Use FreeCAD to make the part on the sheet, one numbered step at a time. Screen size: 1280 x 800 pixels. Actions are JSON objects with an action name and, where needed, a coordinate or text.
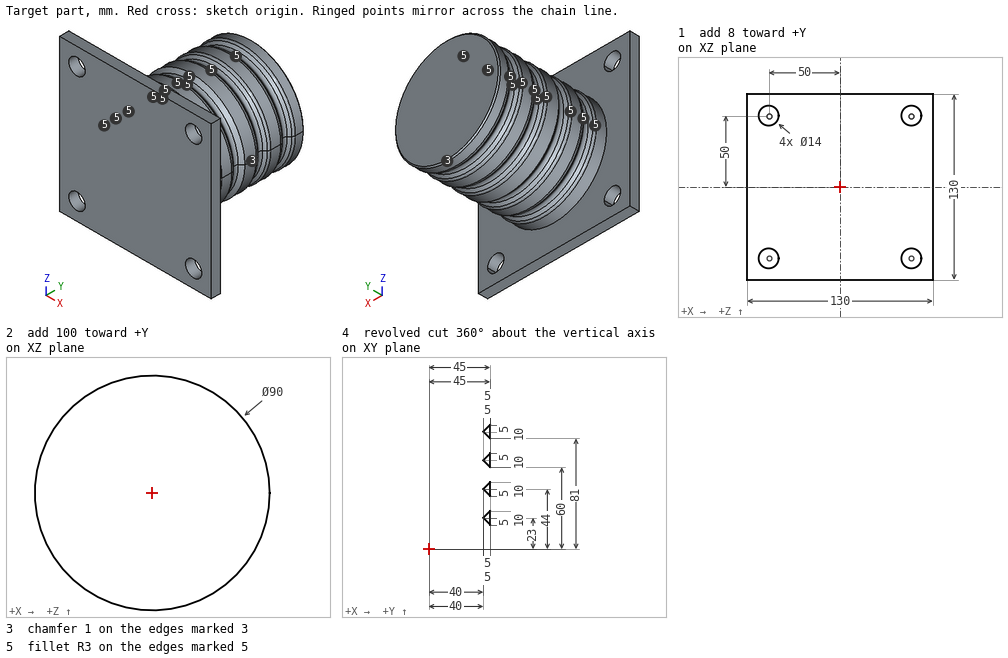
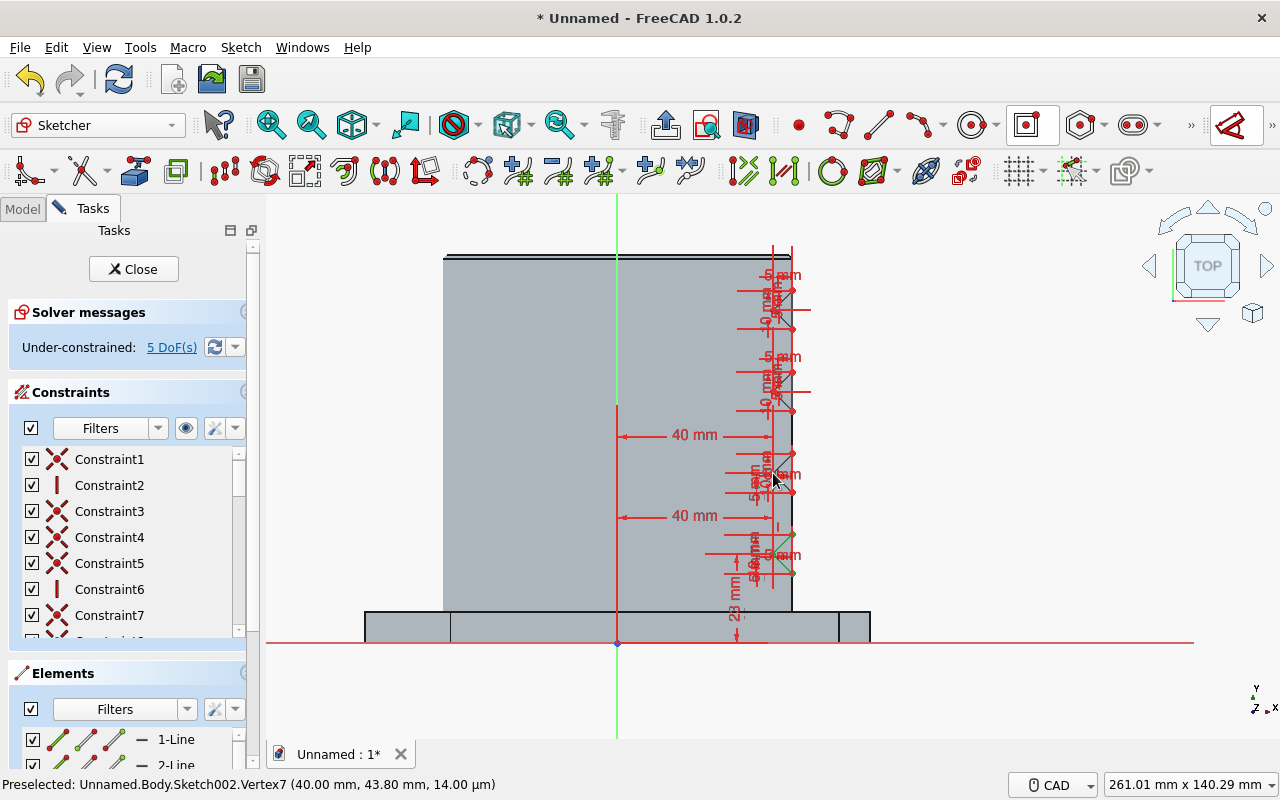
{"action": "left_click", "coordinate": [1258, 126]}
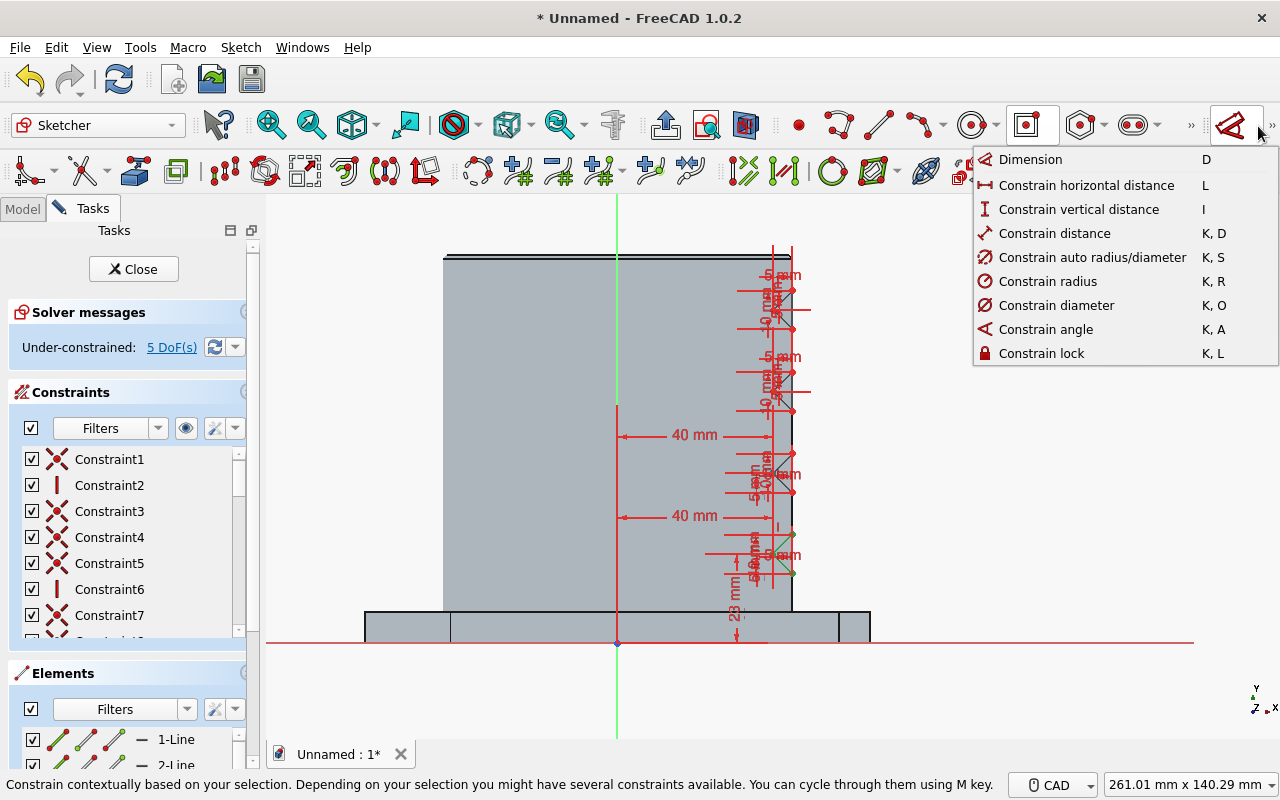
{"action": "left_click", "coordinate": [1126, 209]}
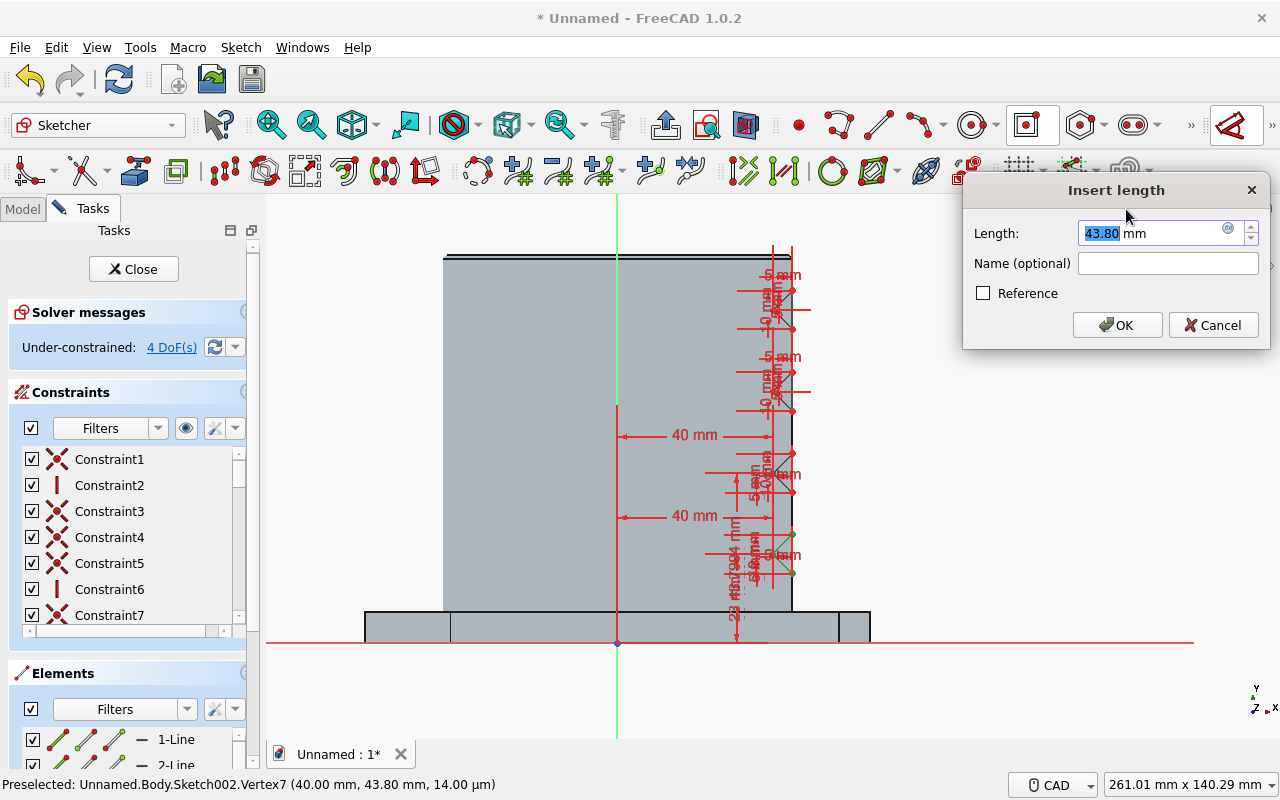
{"action": "type", "text": "44"}
{"action": "key", "text": "Return"}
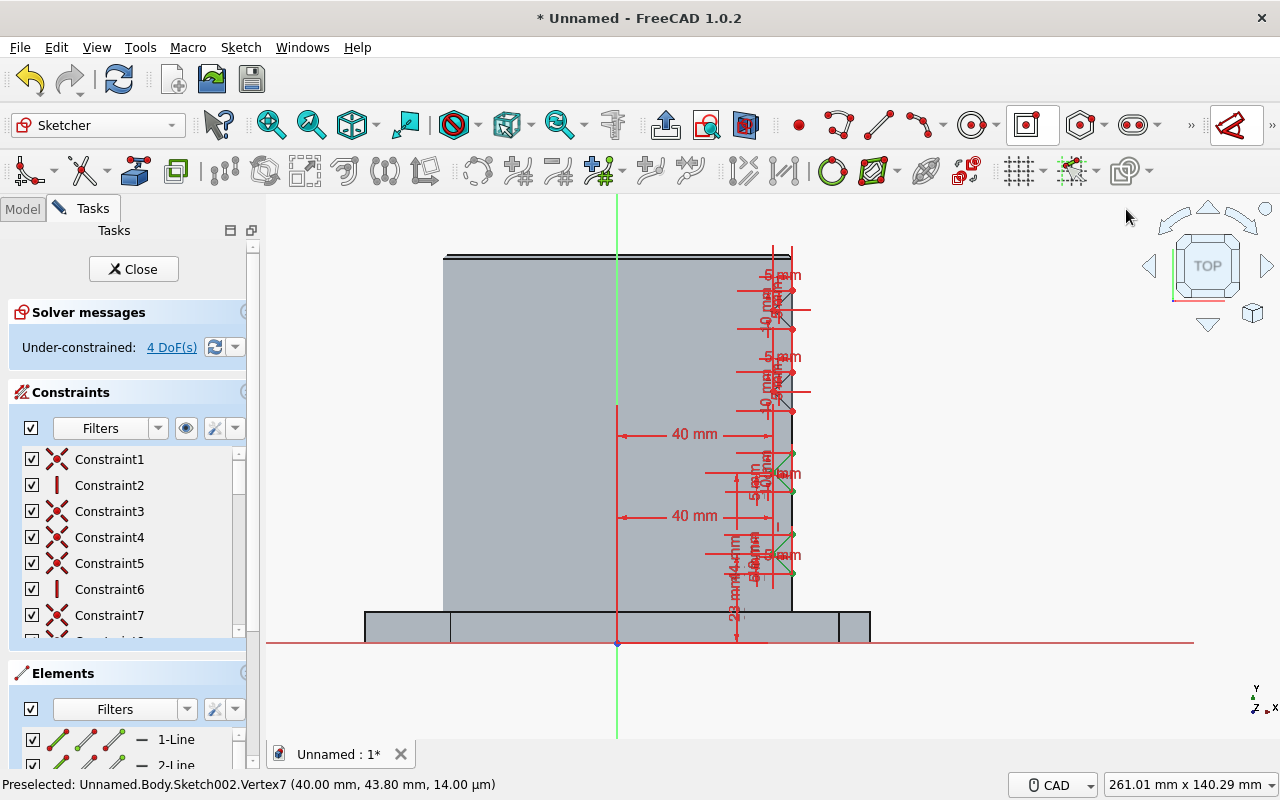
{"action": "left_click", "coordinate": [792, 411]}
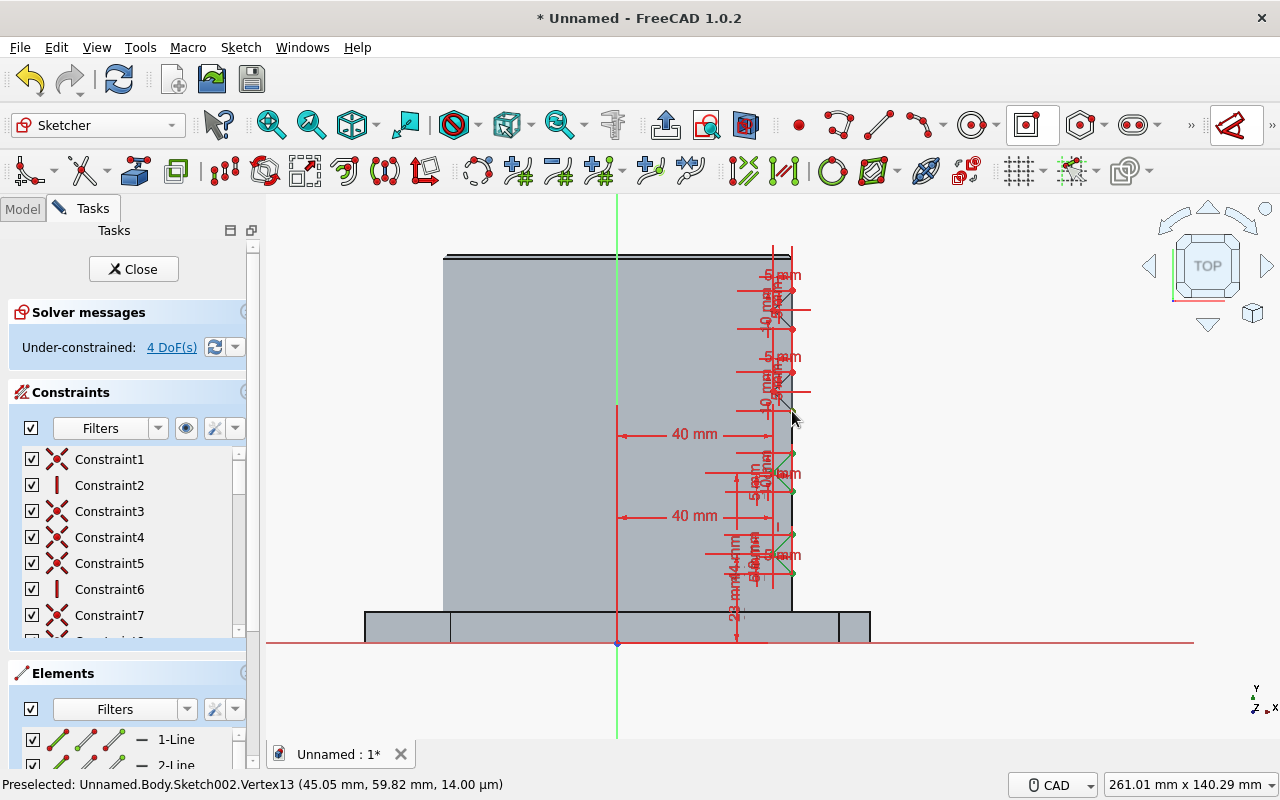
{"action": "left_click", "coordinate": [1258, 126]}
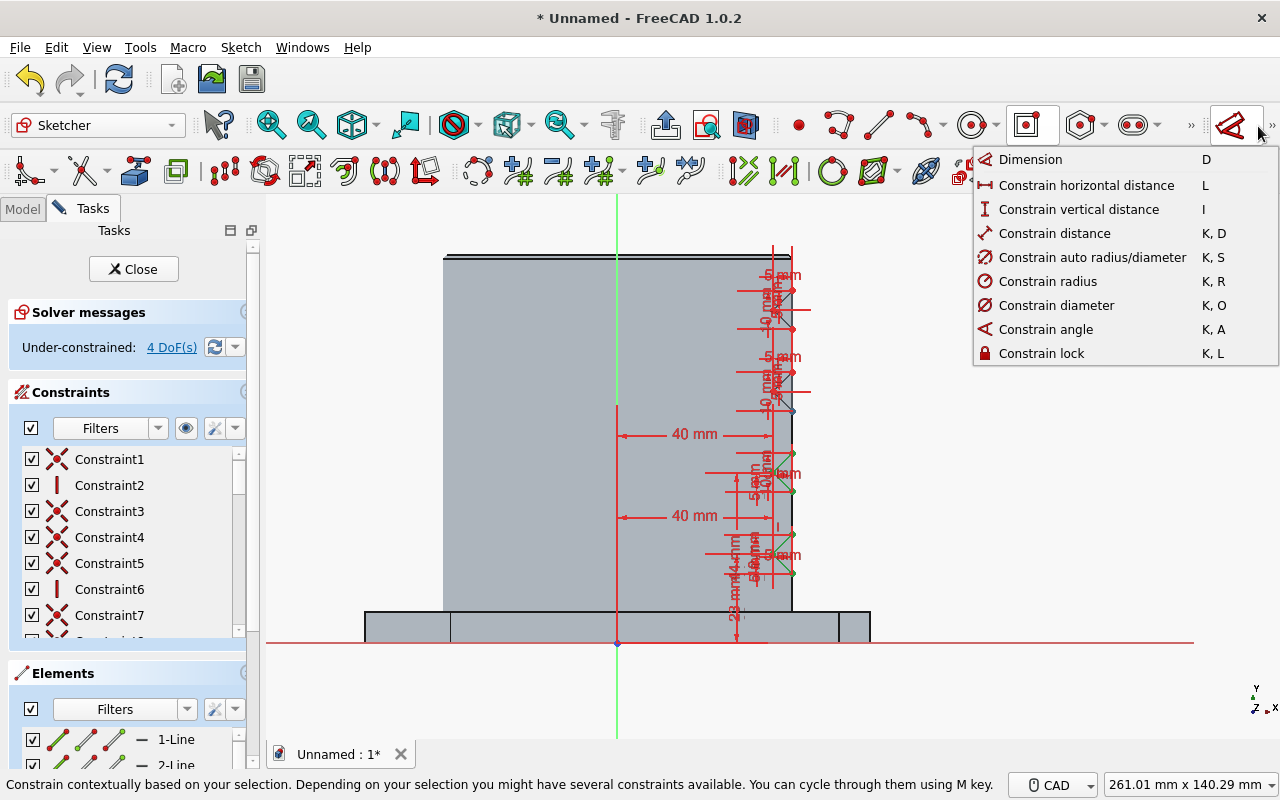
{"action": "left_click", "coordinate": [1126, 185]}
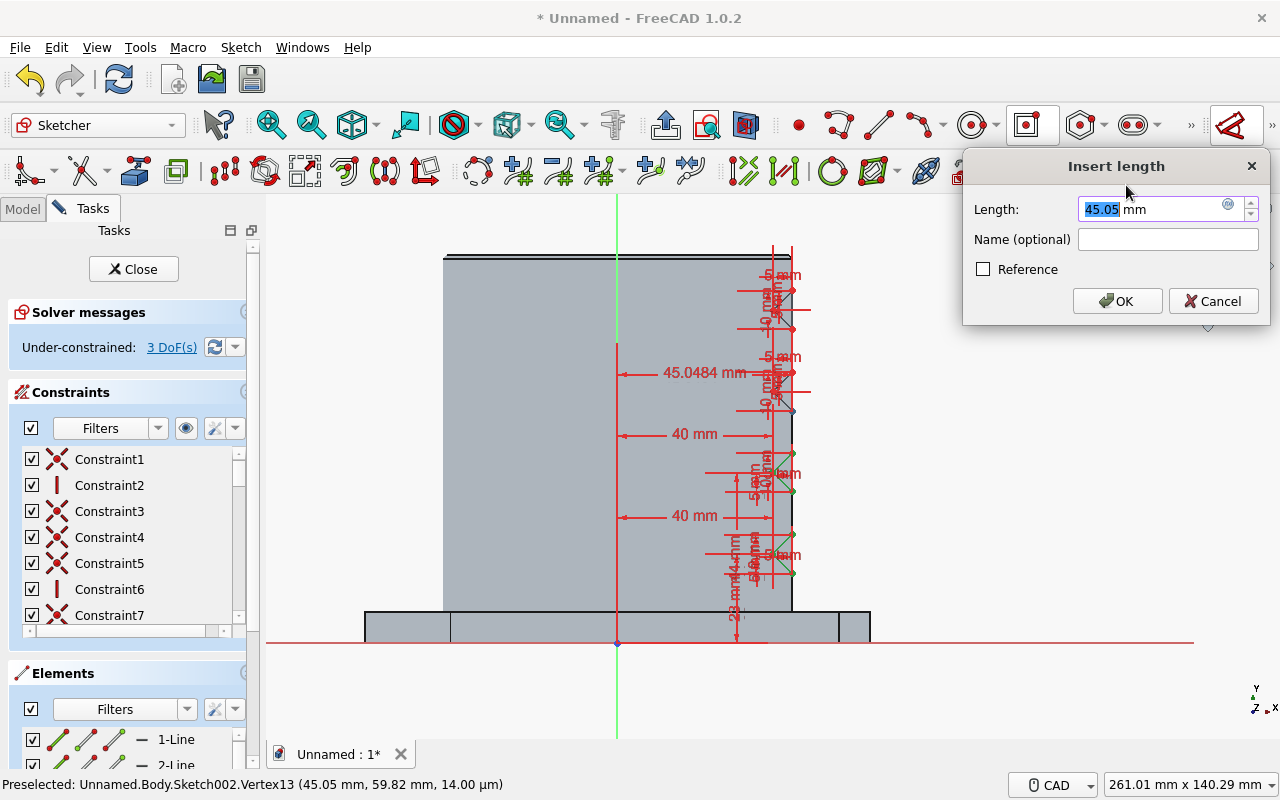
{"action": "type", "text": "45"}
{"action": "key", "text": "Return"}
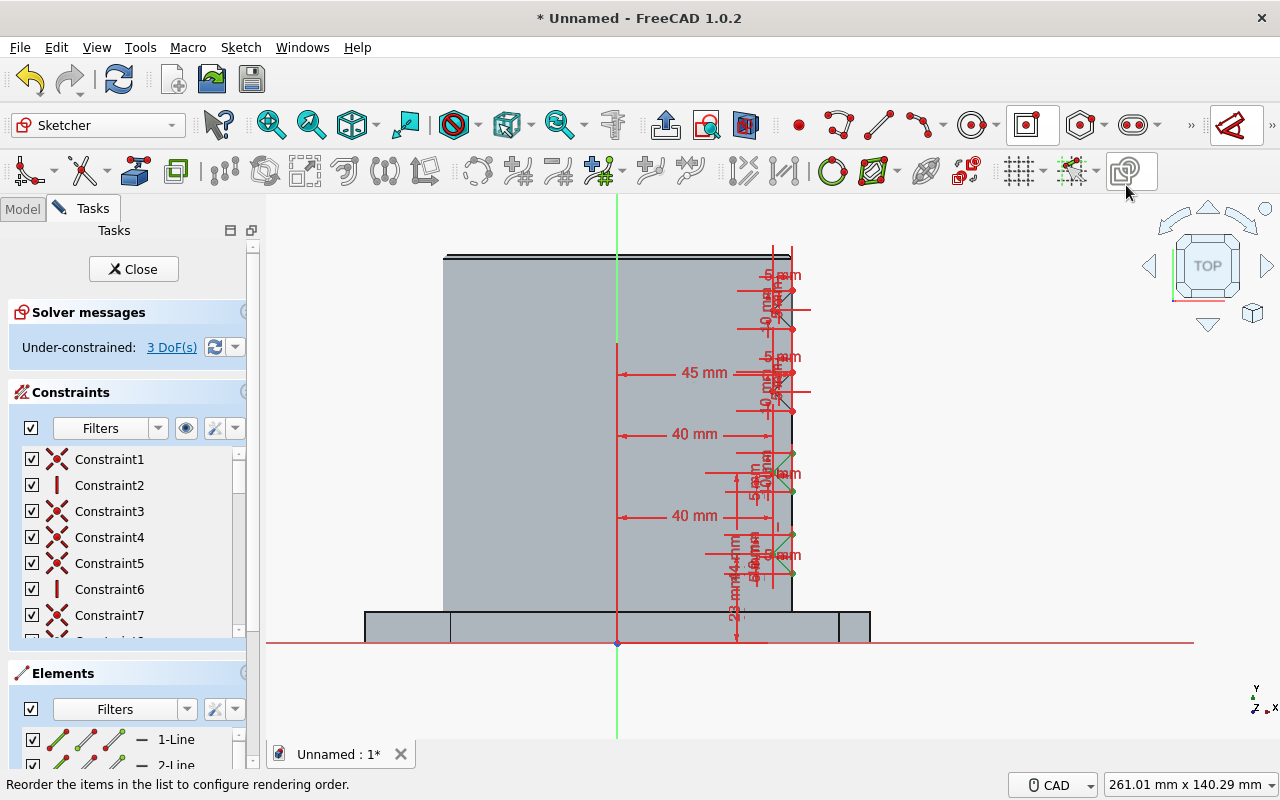
{"action": "left_click", "coordinate": [792, 411]}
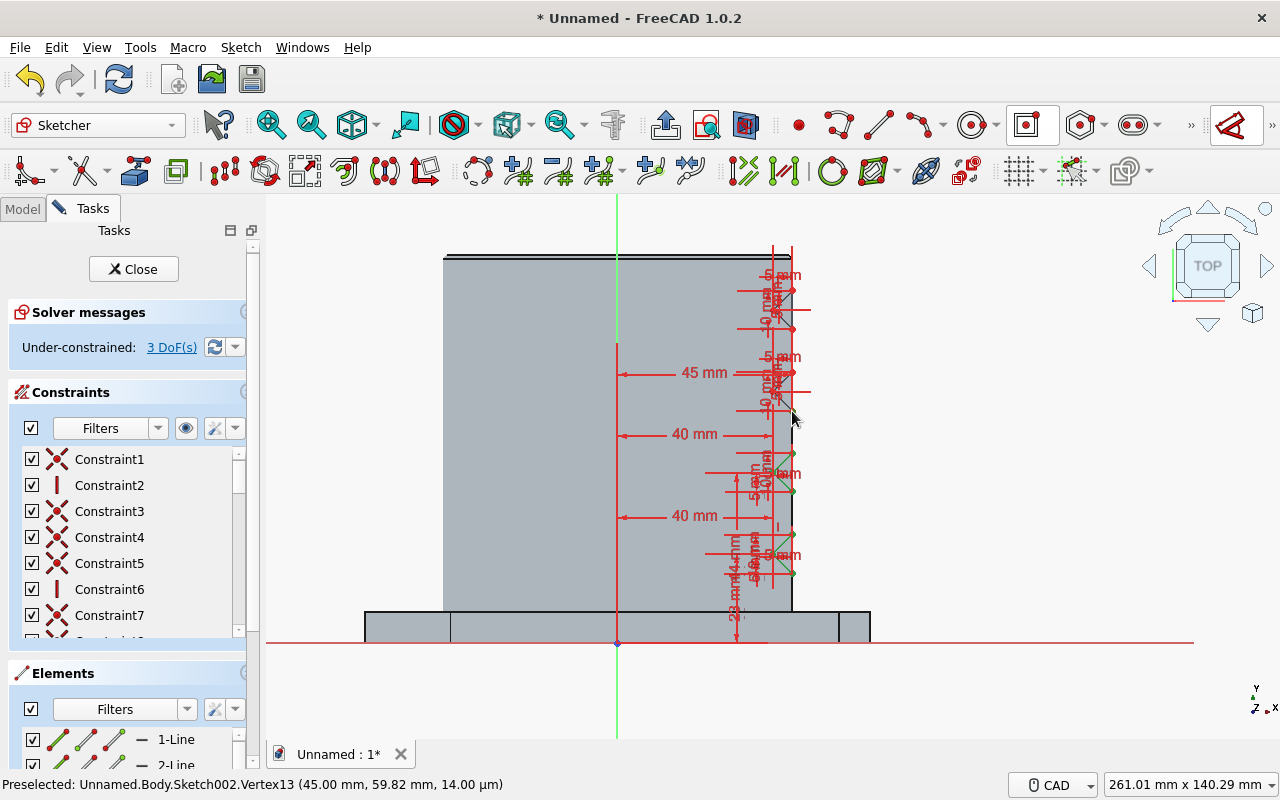
{"action": "left_click", "coordinate": [1258, 126]}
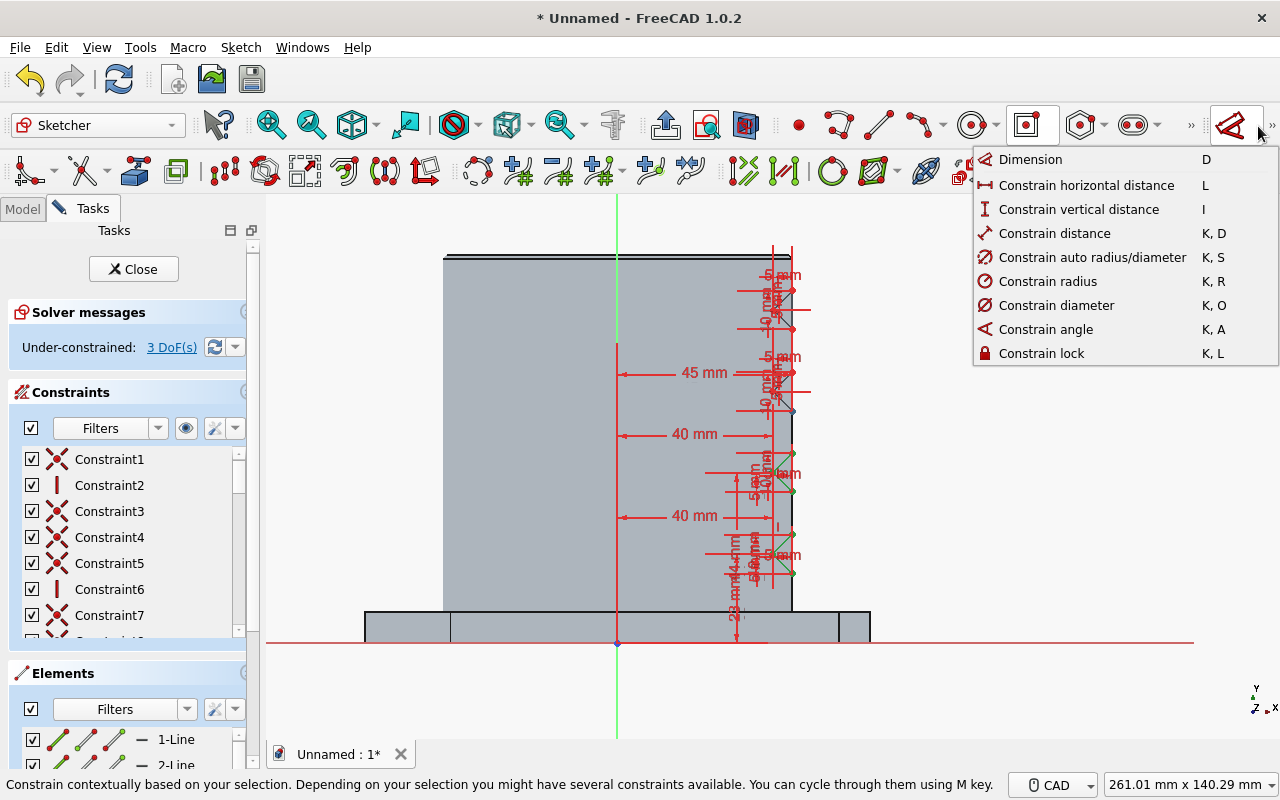
{"action": "left_click", "coordinate": [1126, 209]}